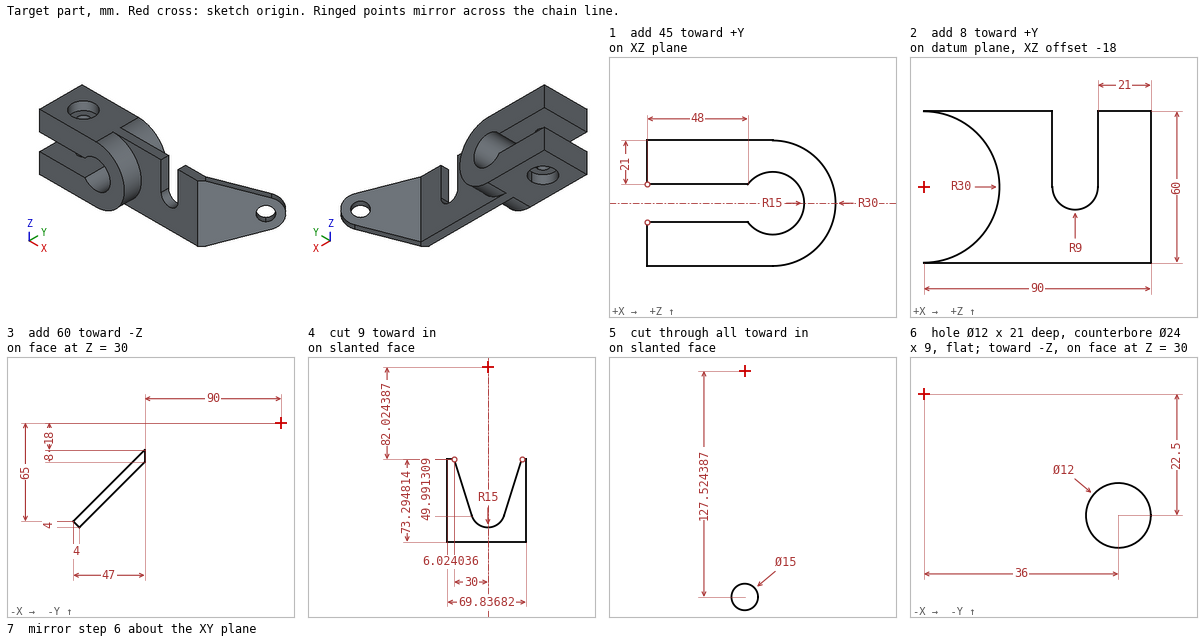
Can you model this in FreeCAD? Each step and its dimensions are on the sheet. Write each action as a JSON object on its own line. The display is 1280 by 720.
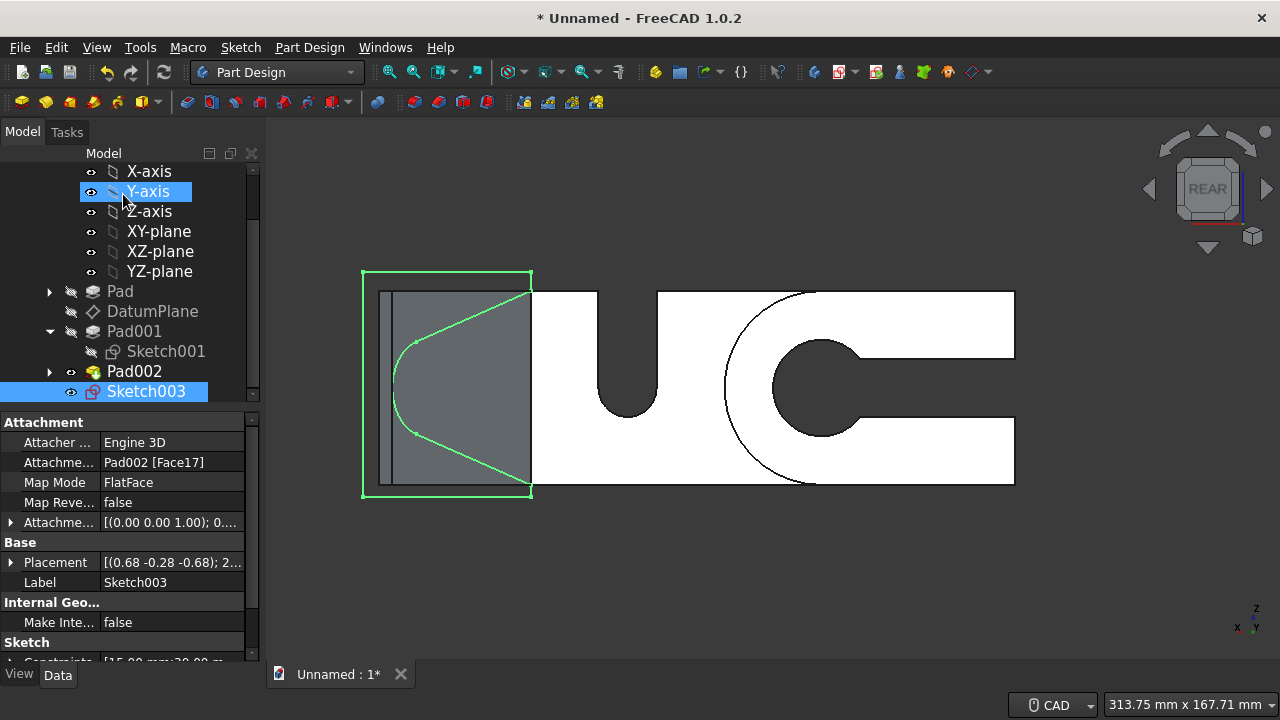
{"action": "left_click", "coordinate": [188, 102]}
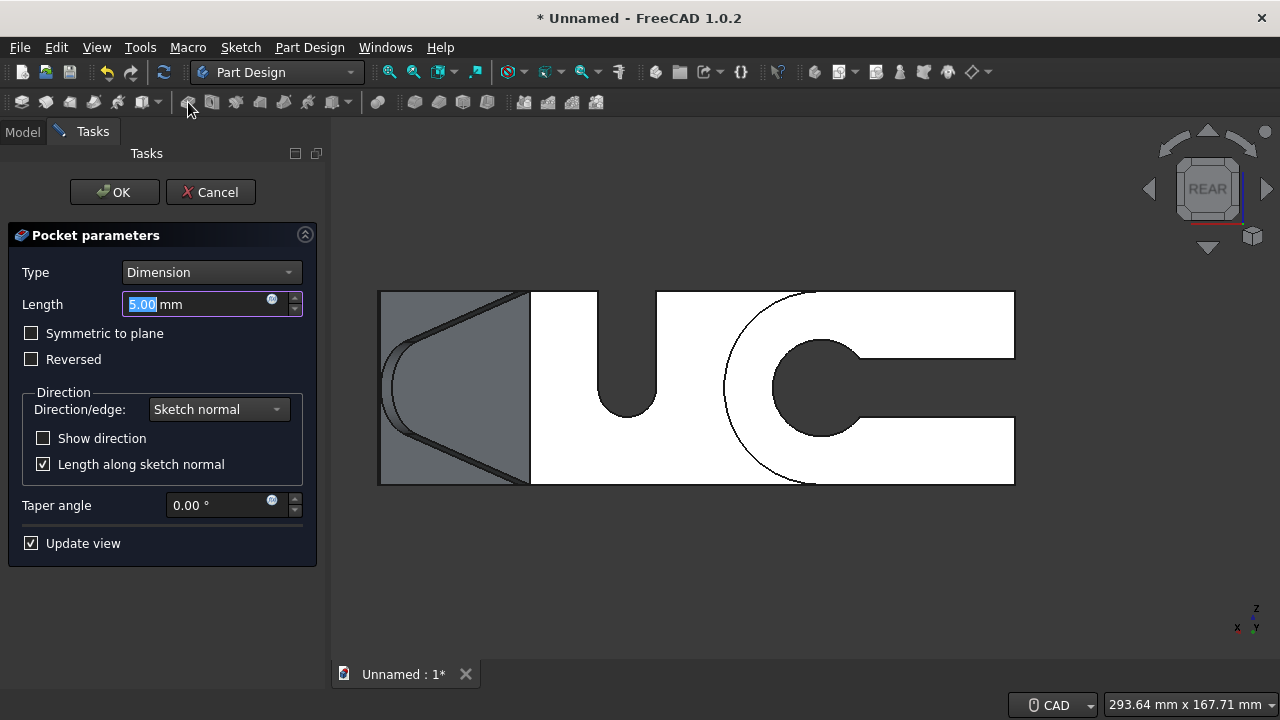
{"action": "type", "text": "9"}
{"action": "key", "text": "Tab"}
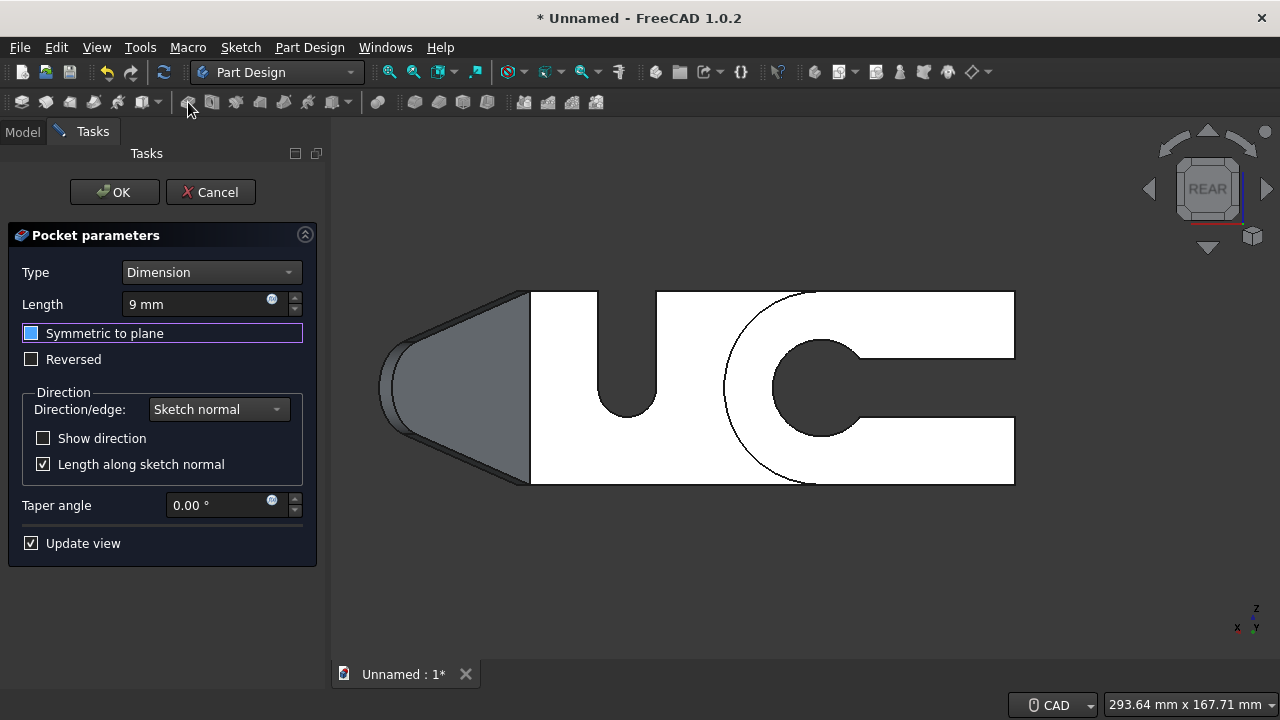
{"action": "left_click", "coordinate": [115, 192]}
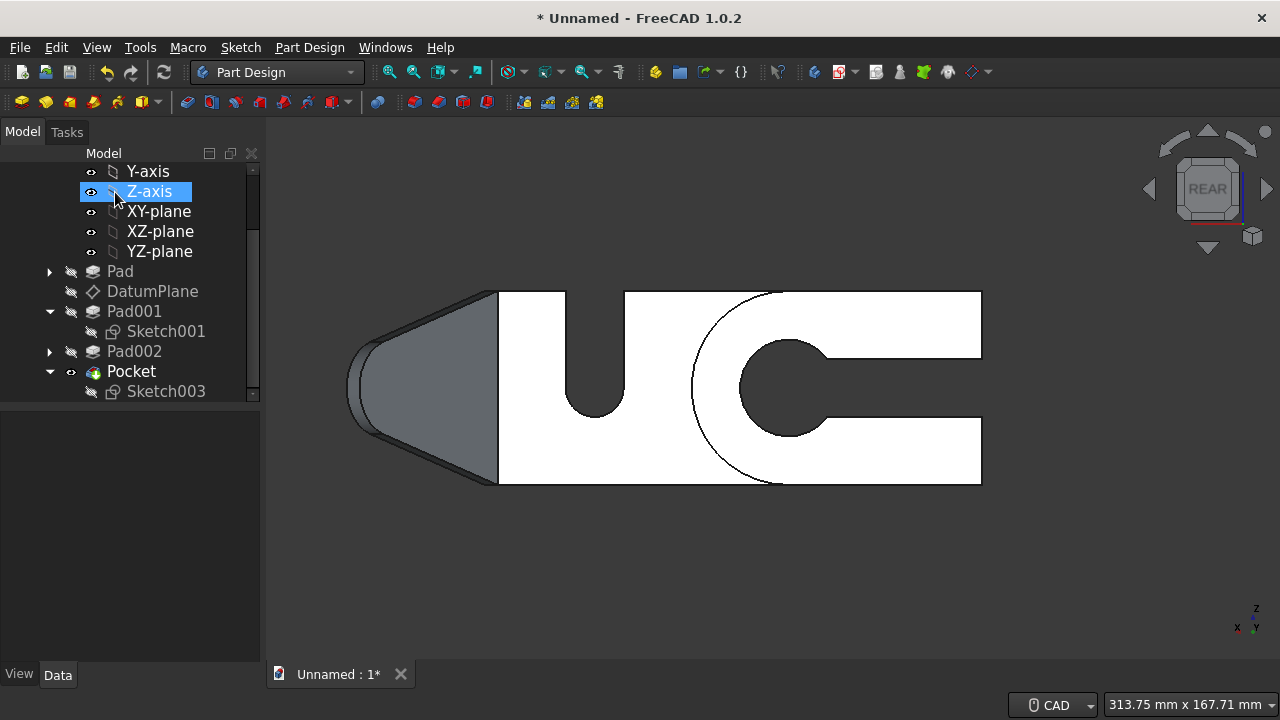
{"action": "left_click", "coordinate": [448, 387]}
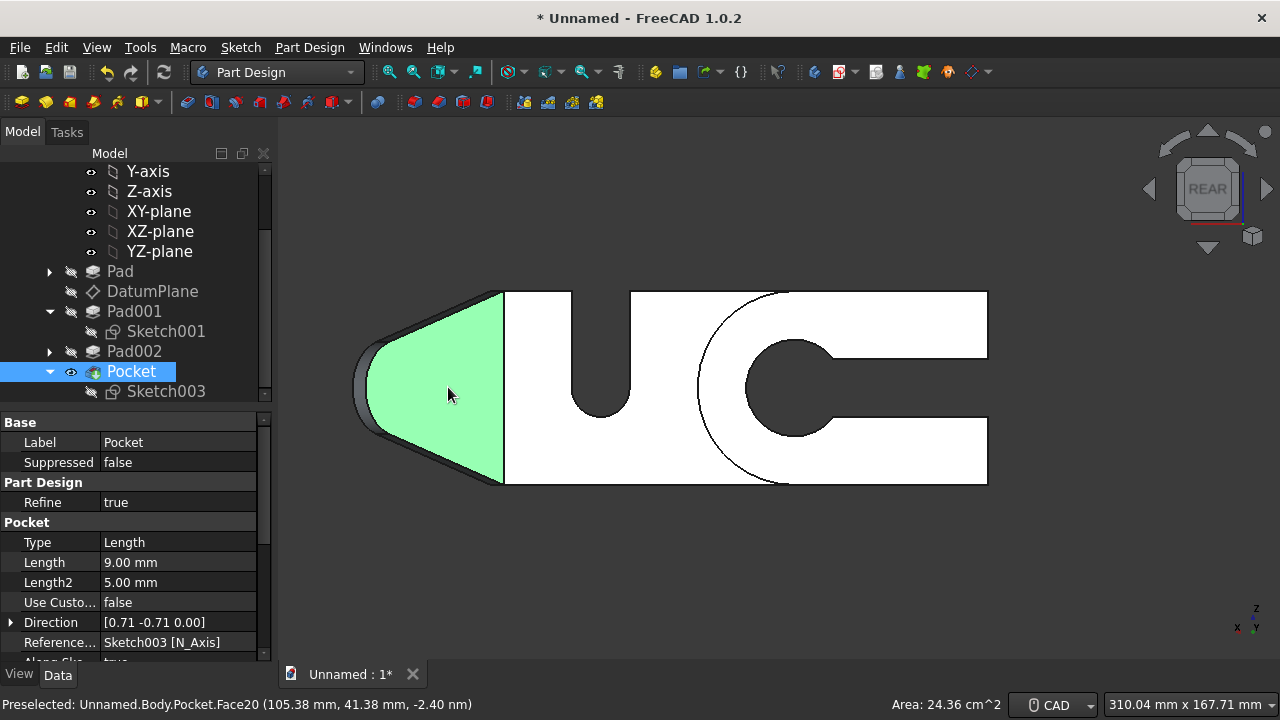
{"action": "left_click", "coordinate": [840, 72]}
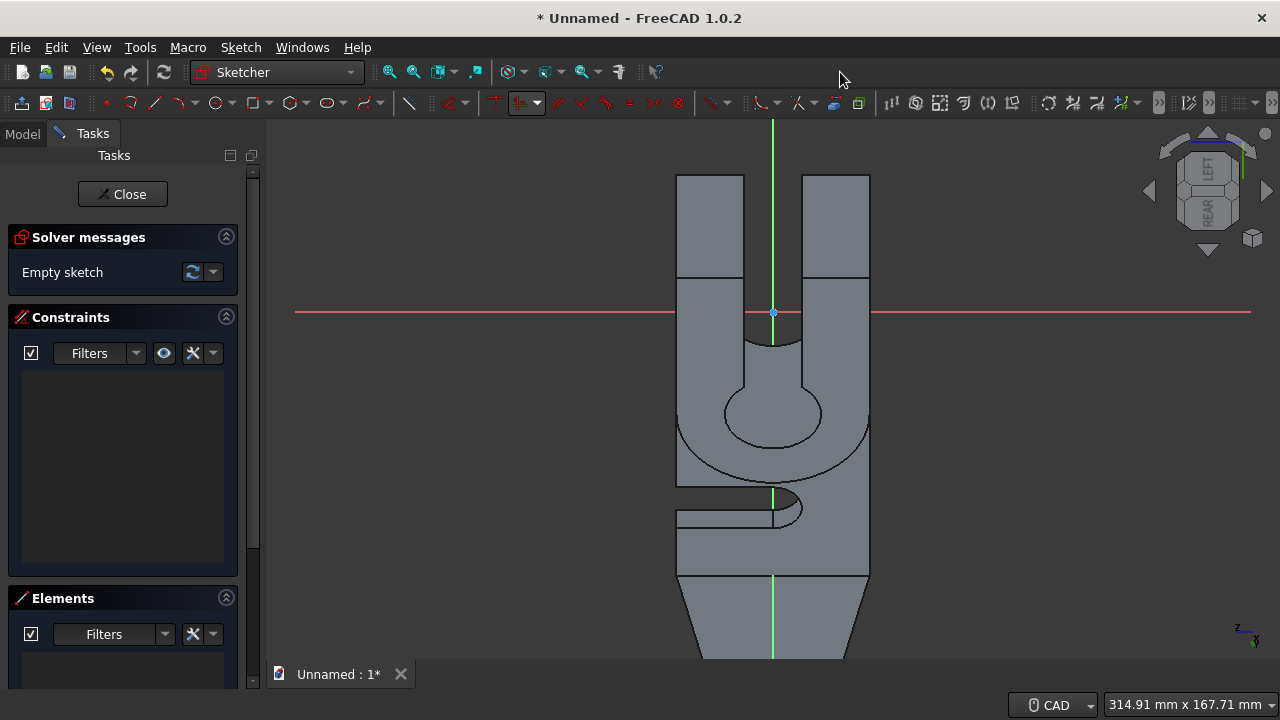
{"action": "scroll", "coordinate": [704, 389], "scroll_direction": "down", "scroll_amount": 5}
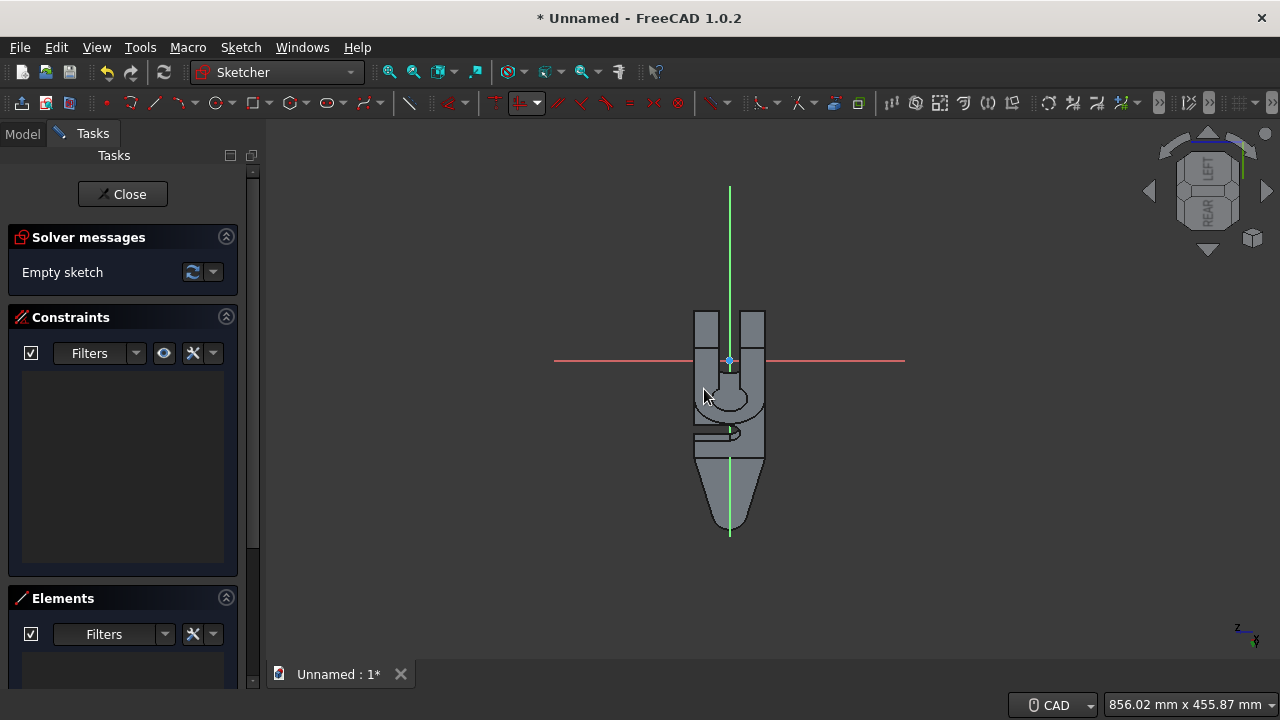
{"action": "scroll", "coordinate": [731, 518], "scroll_direction": "up", "scroll_amount": 15}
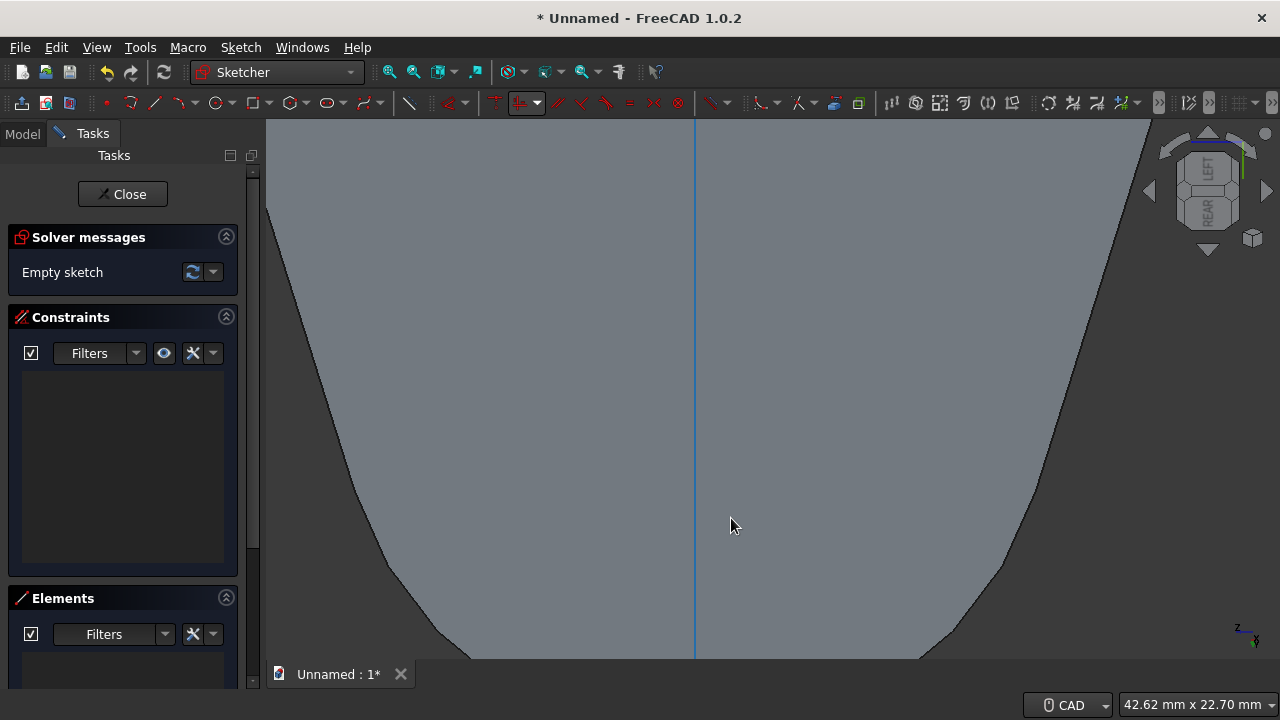
{"action": "key", "text": "g c"}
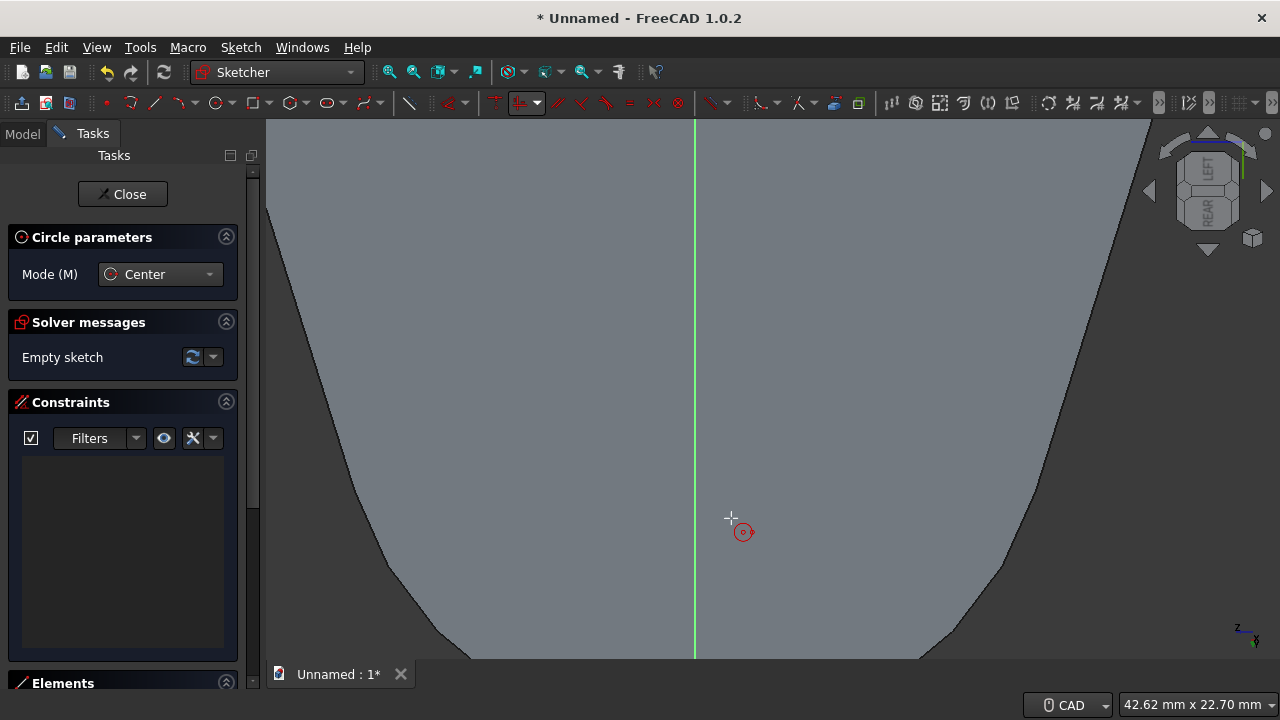
{"action": "left_click", "coordinate": [695, 384]}
{"action": "mouse_move", "coordinate": [821, 258]}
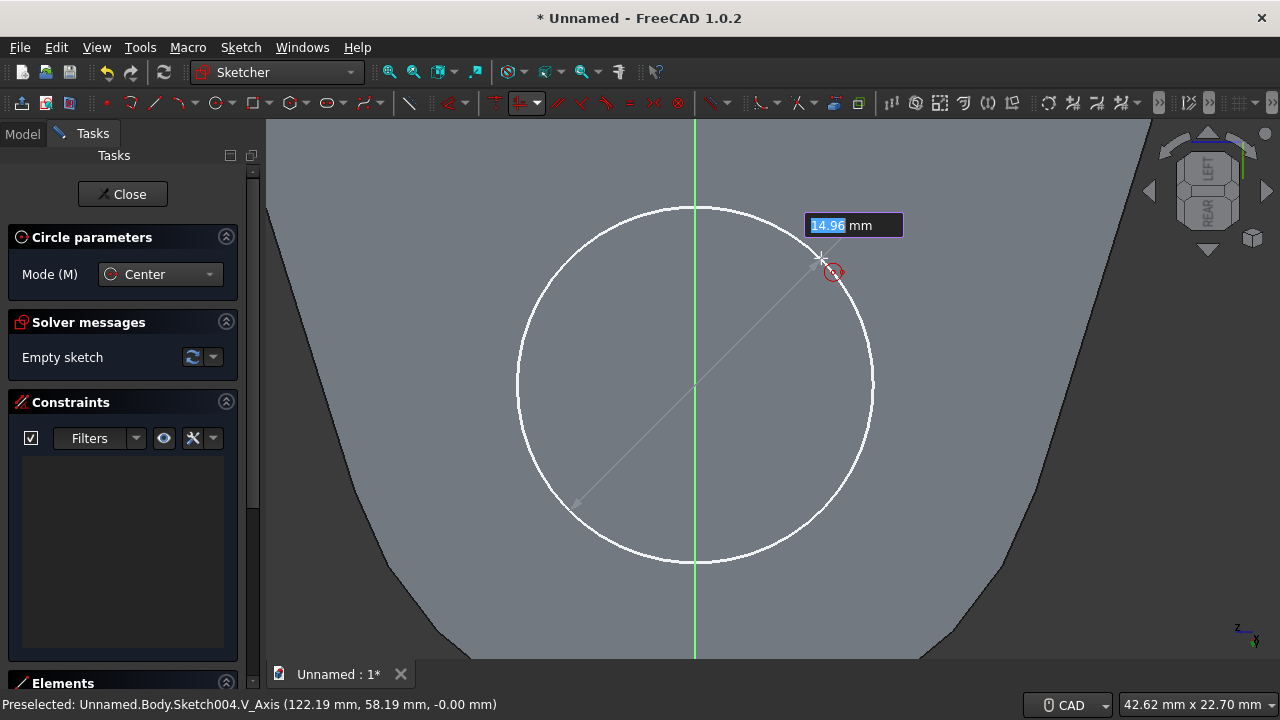
{"action": "type", "text": "15"}
{"action": "key", "text": "Return"}
{"action": "key", "text": "Escape"}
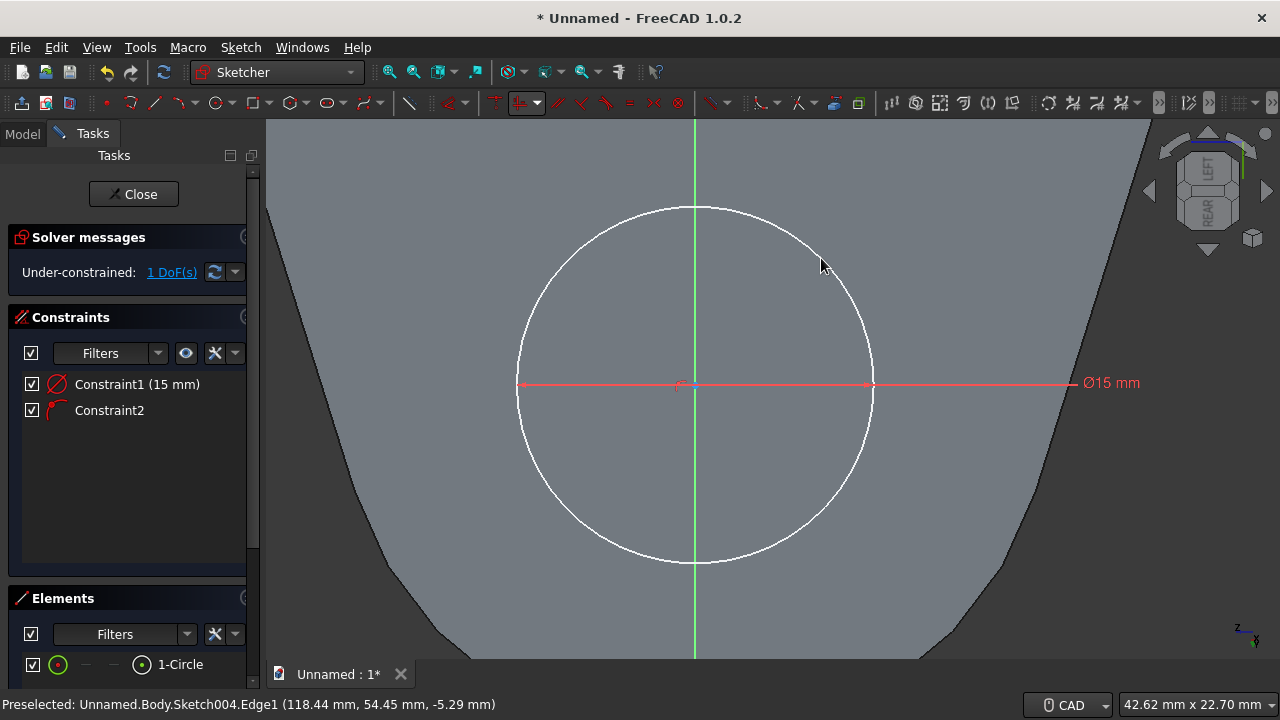
{"action": "left_click", "coordinate": [448, 104]}